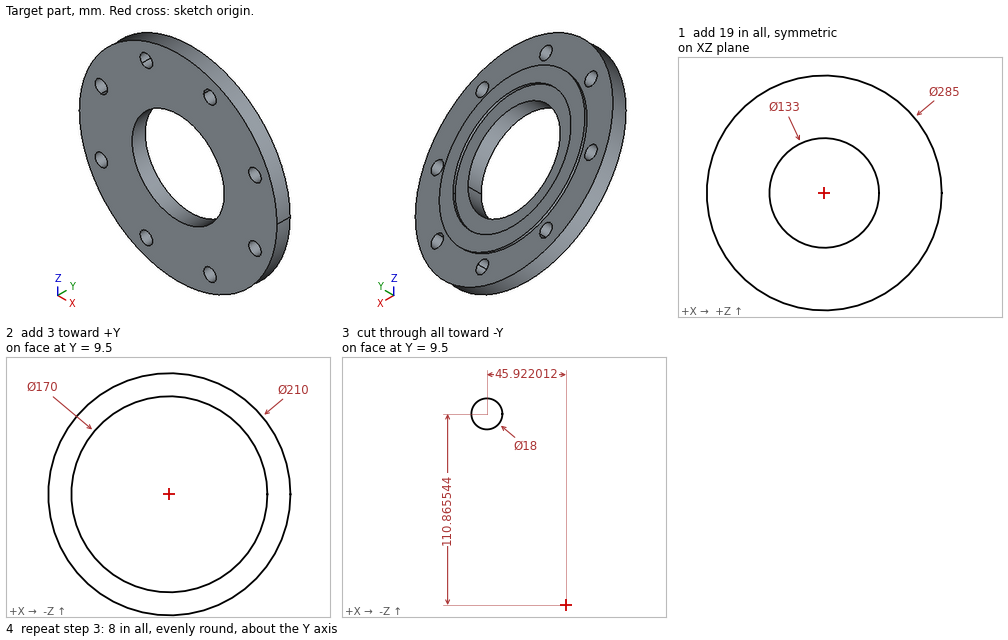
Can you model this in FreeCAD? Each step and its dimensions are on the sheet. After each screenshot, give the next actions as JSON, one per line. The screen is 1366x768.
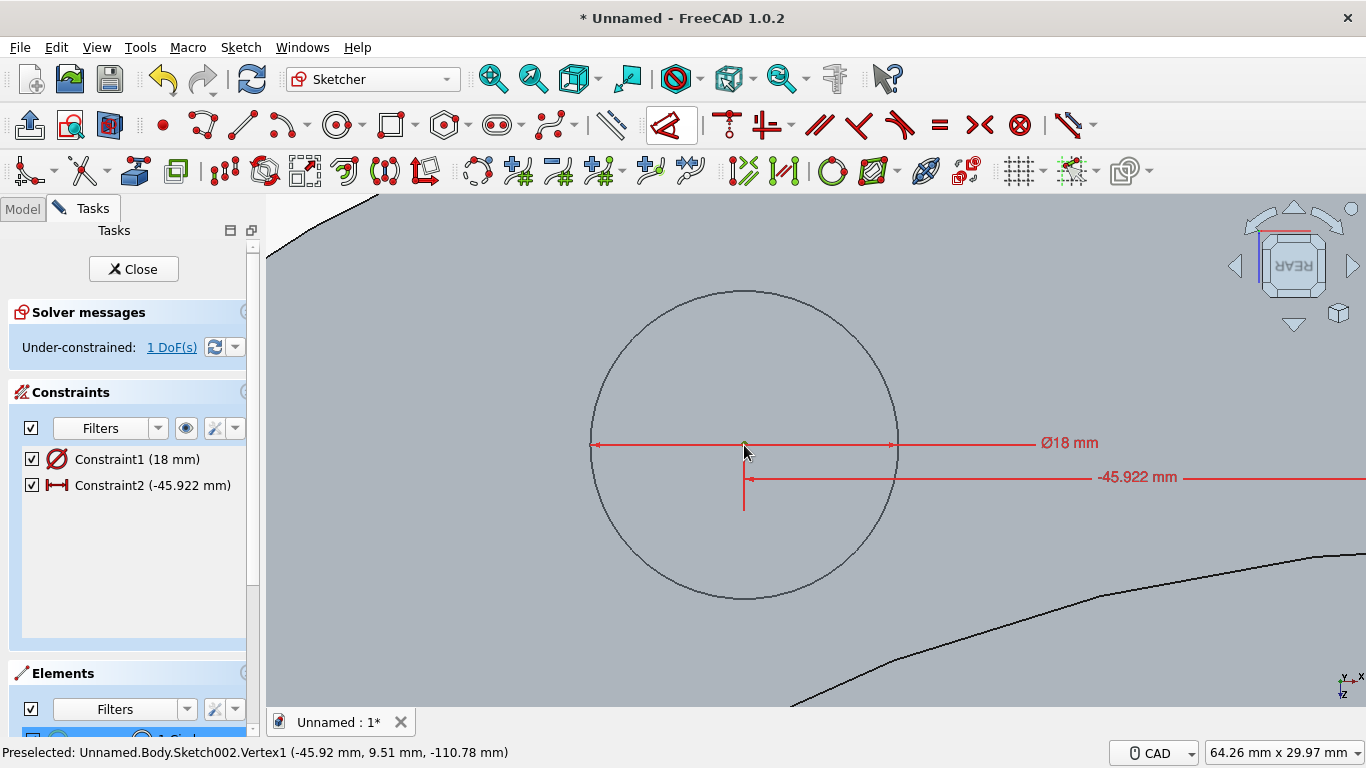
{"action": "key", "text": "i"}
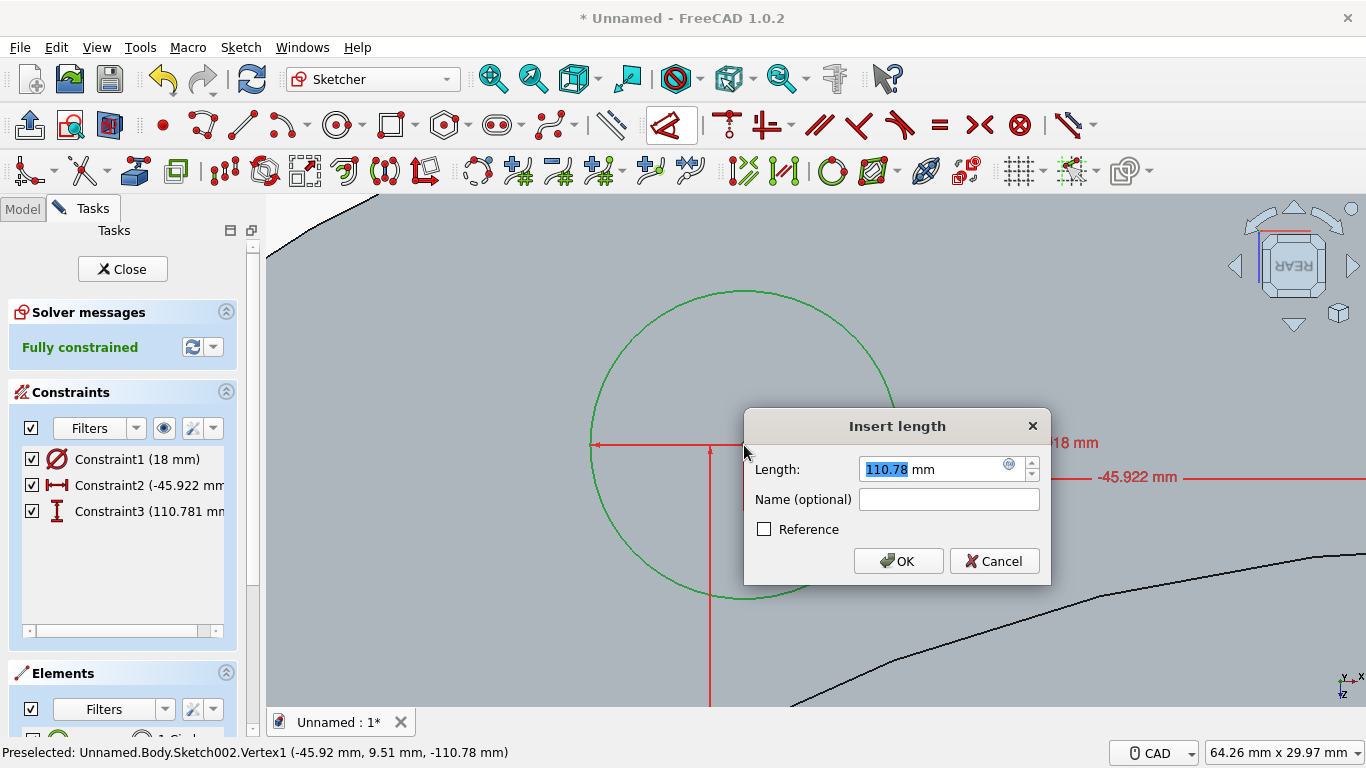
{"action": "type", "text": "110.865544"}
{"action": "key", "text": "Return"}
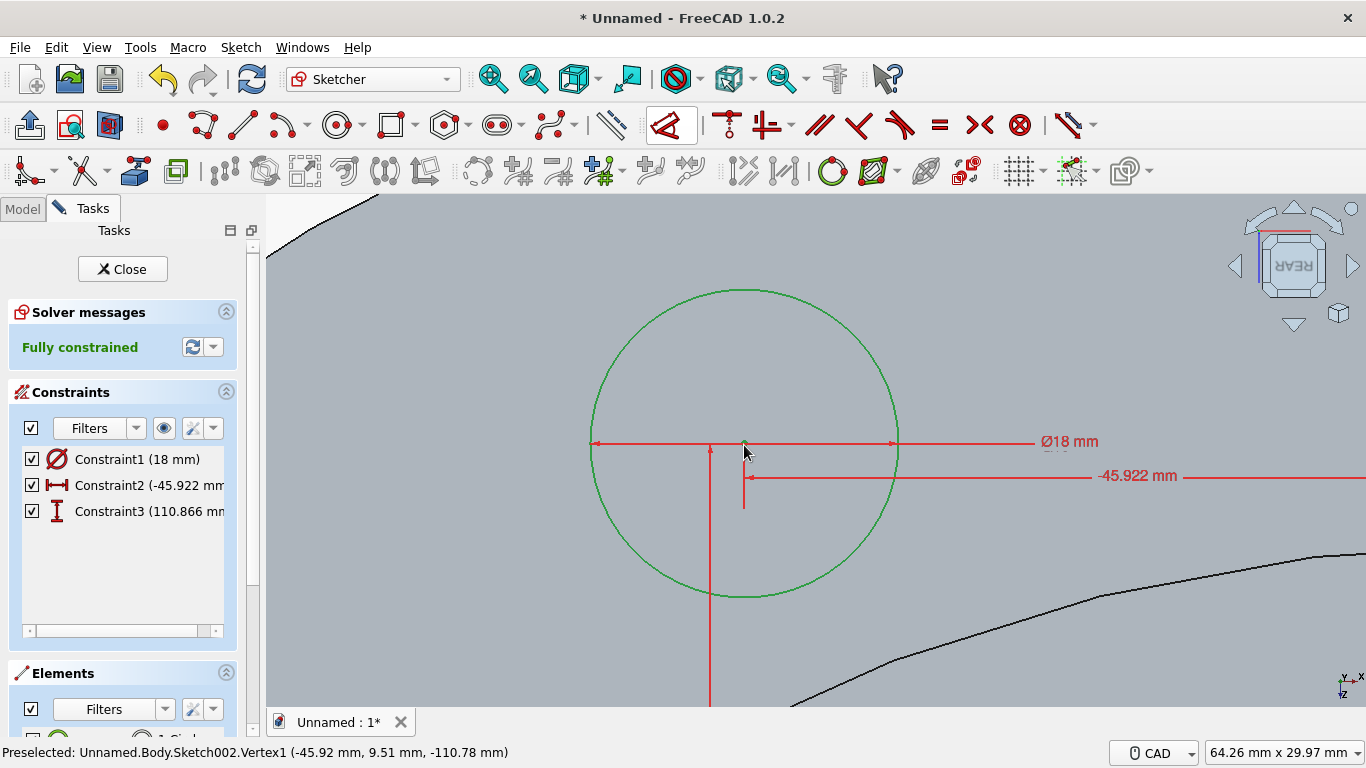
{"action": "left_click", "coordinate": [123, 269]}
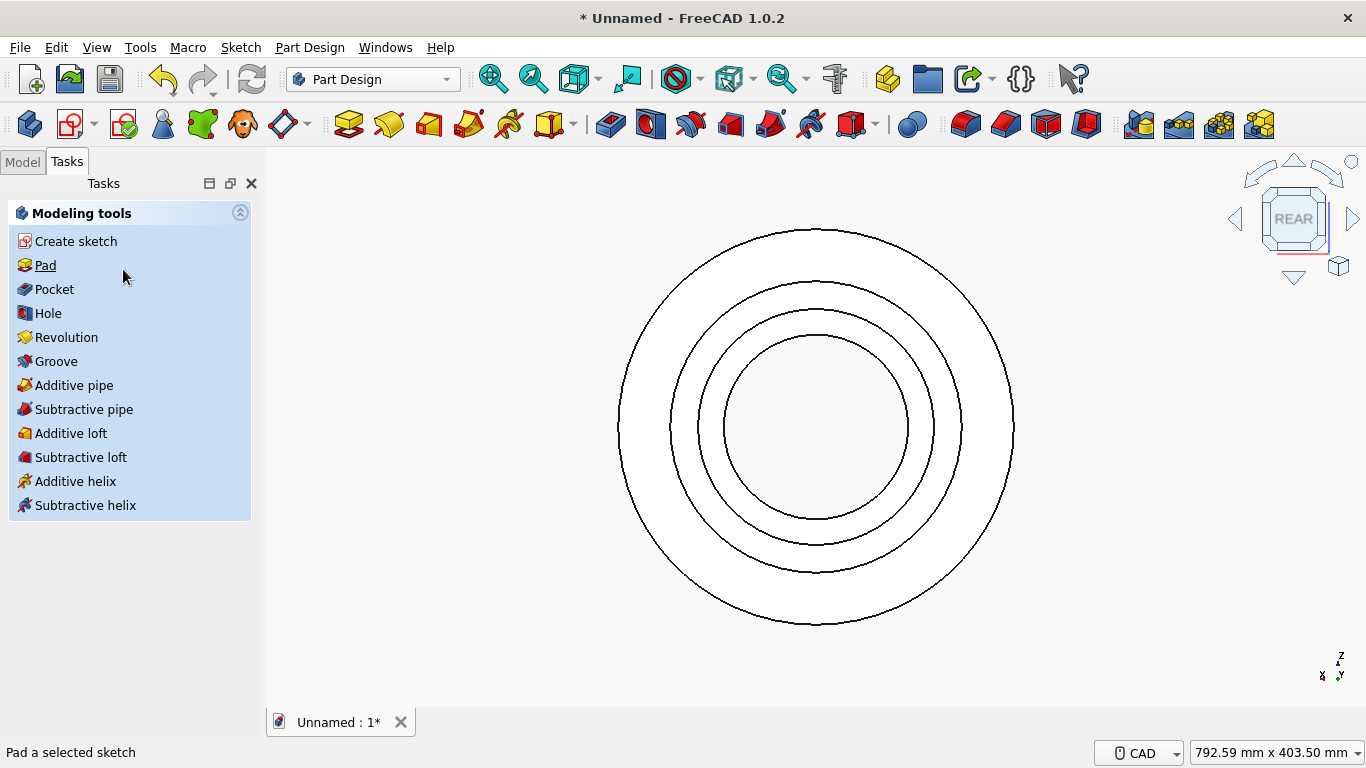
{"action": "left_click", "coordinate": [612, 124]}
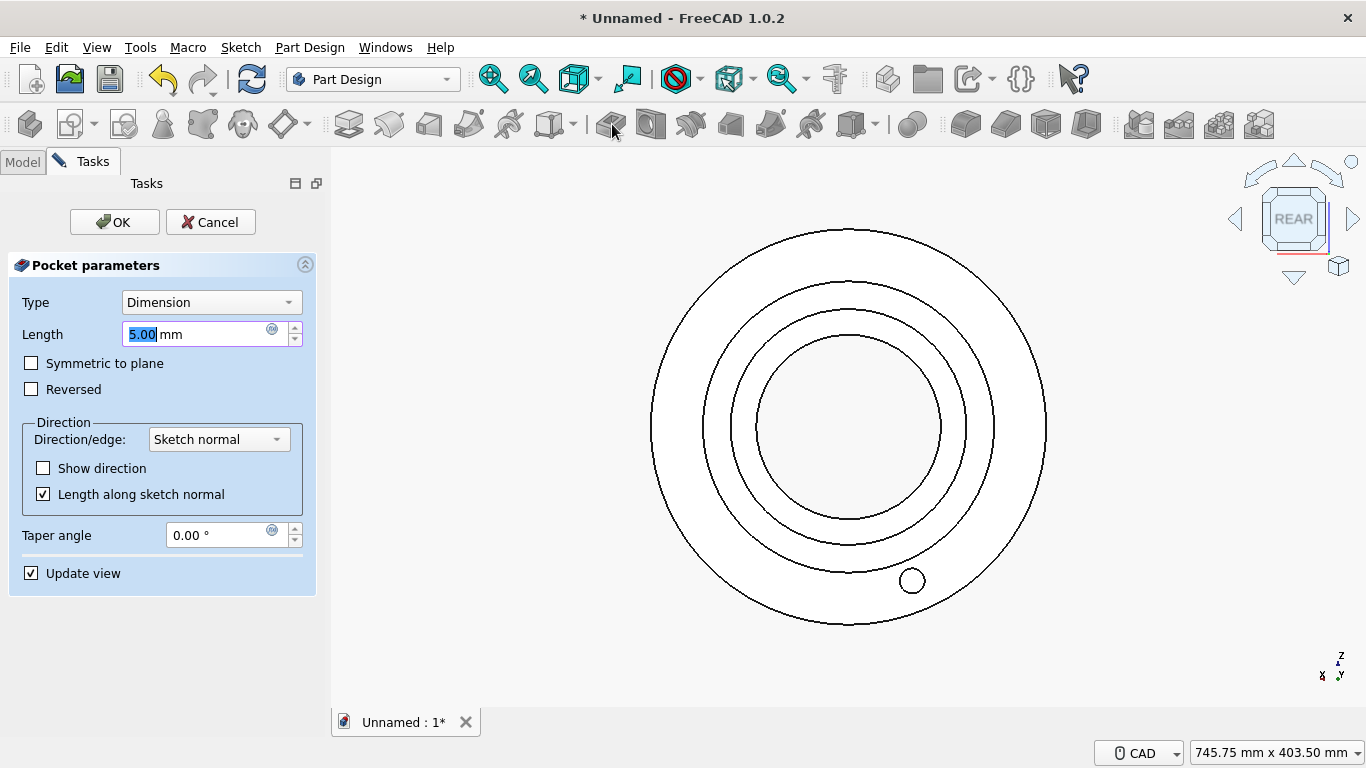
{"action": "left_click", "coordinate": [212, 302]}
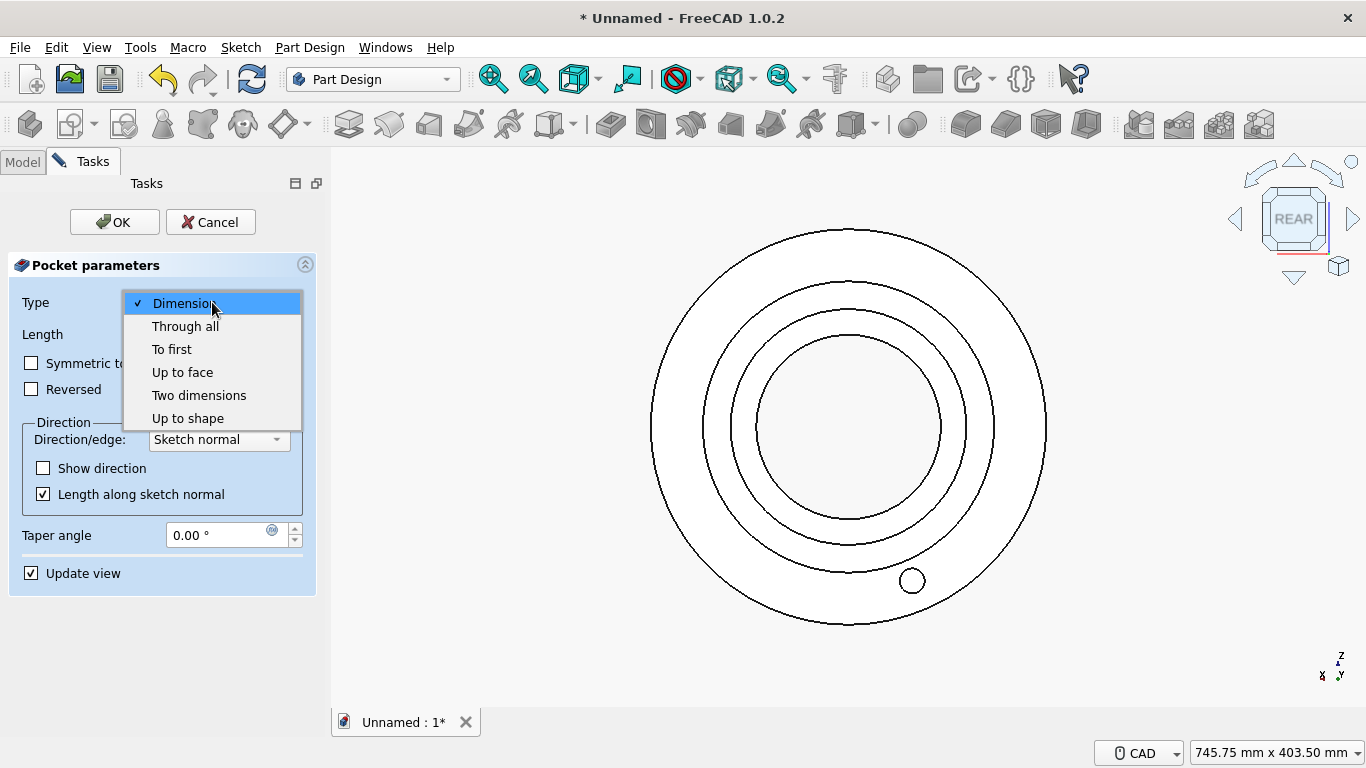
{"action": "left_click", "coordinate": [212, 326]}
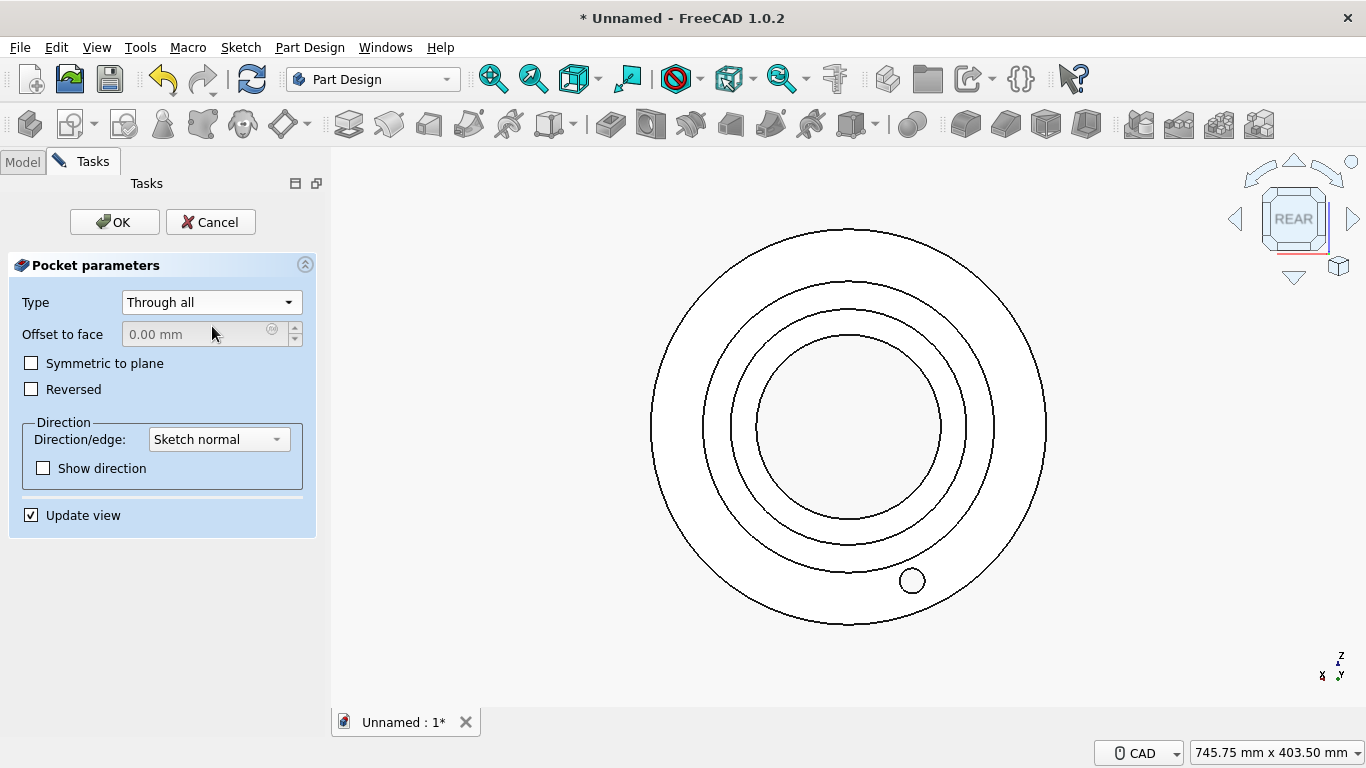
{"action": "left_click", "coordinate": [115, 222]}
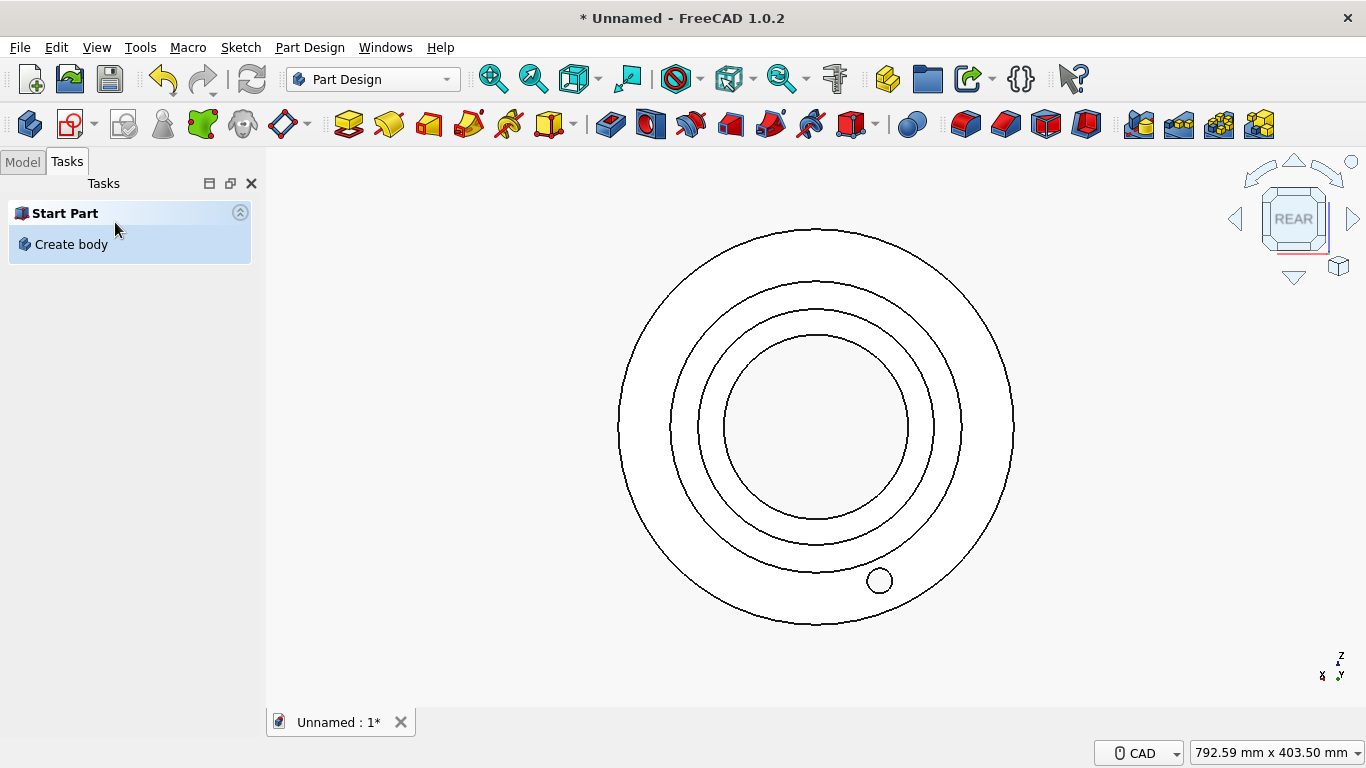
{"action": "left_click", "coordinate": [23, 161]}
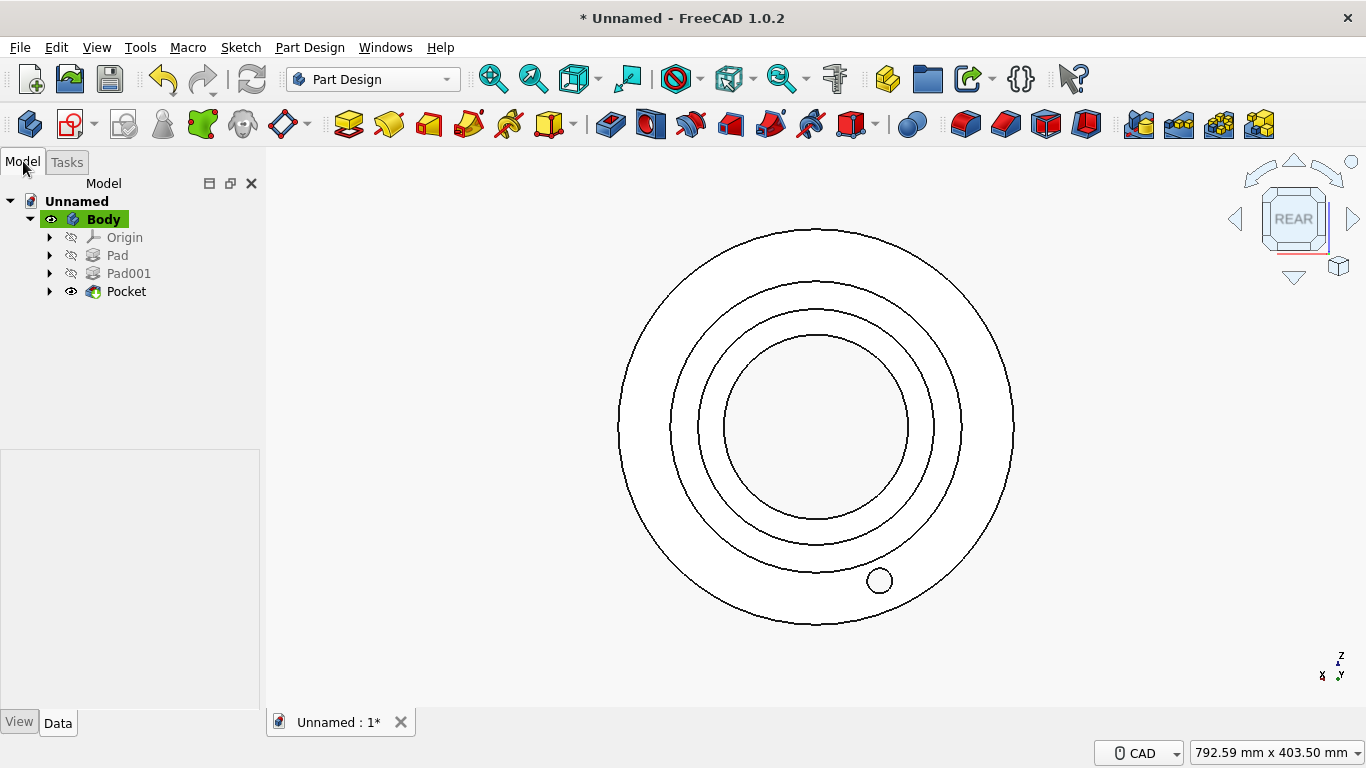
{"action": "left_click", "coordinate": [116, 291]}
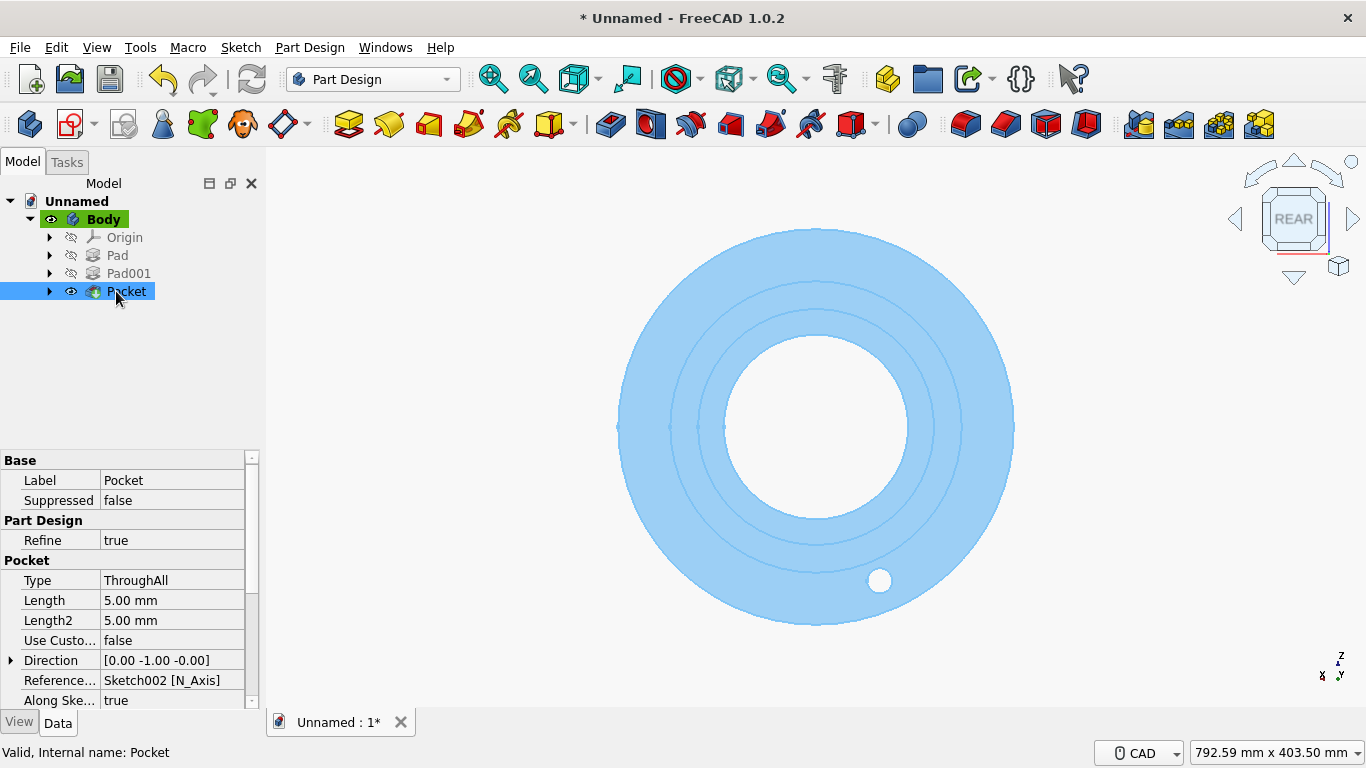
{"action": "left_click", "coordinate": [1220, 124]}